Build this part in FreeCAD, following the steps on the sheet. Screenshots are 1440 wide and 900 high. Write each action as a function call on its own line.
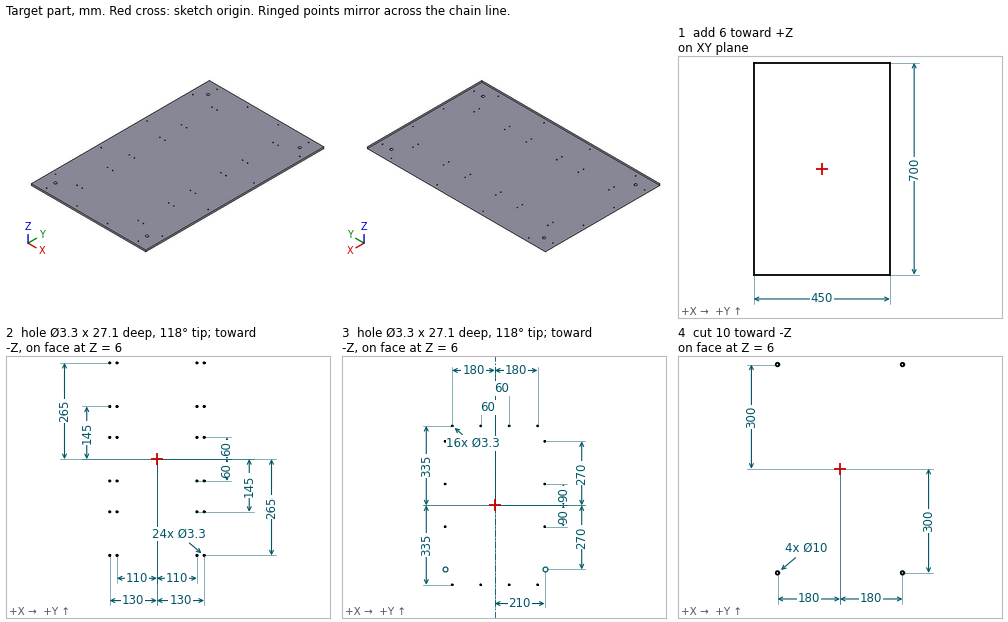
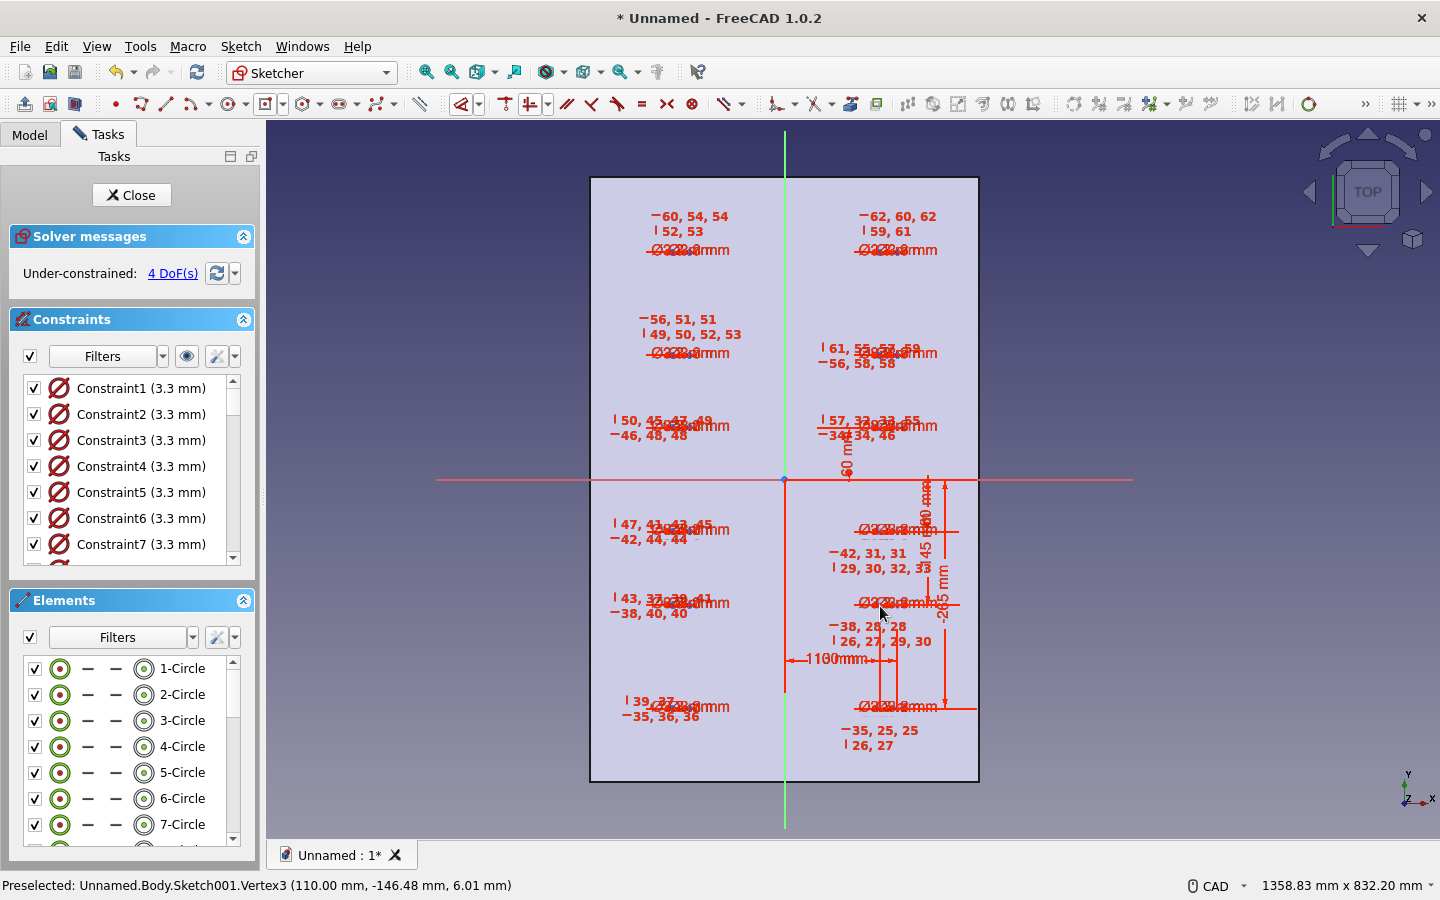
click(672, 709)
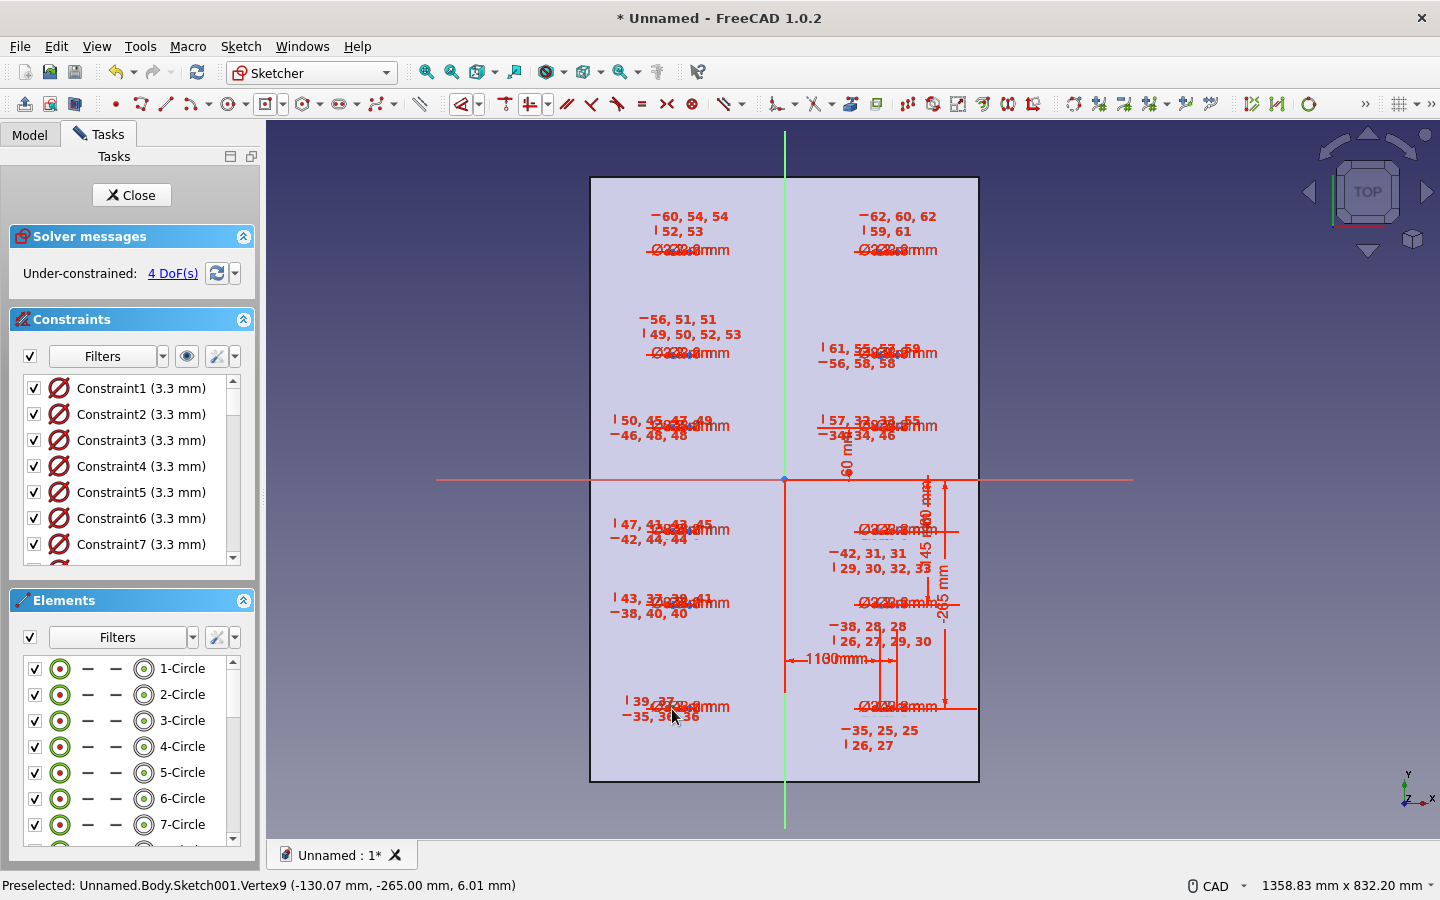
click(478, 104)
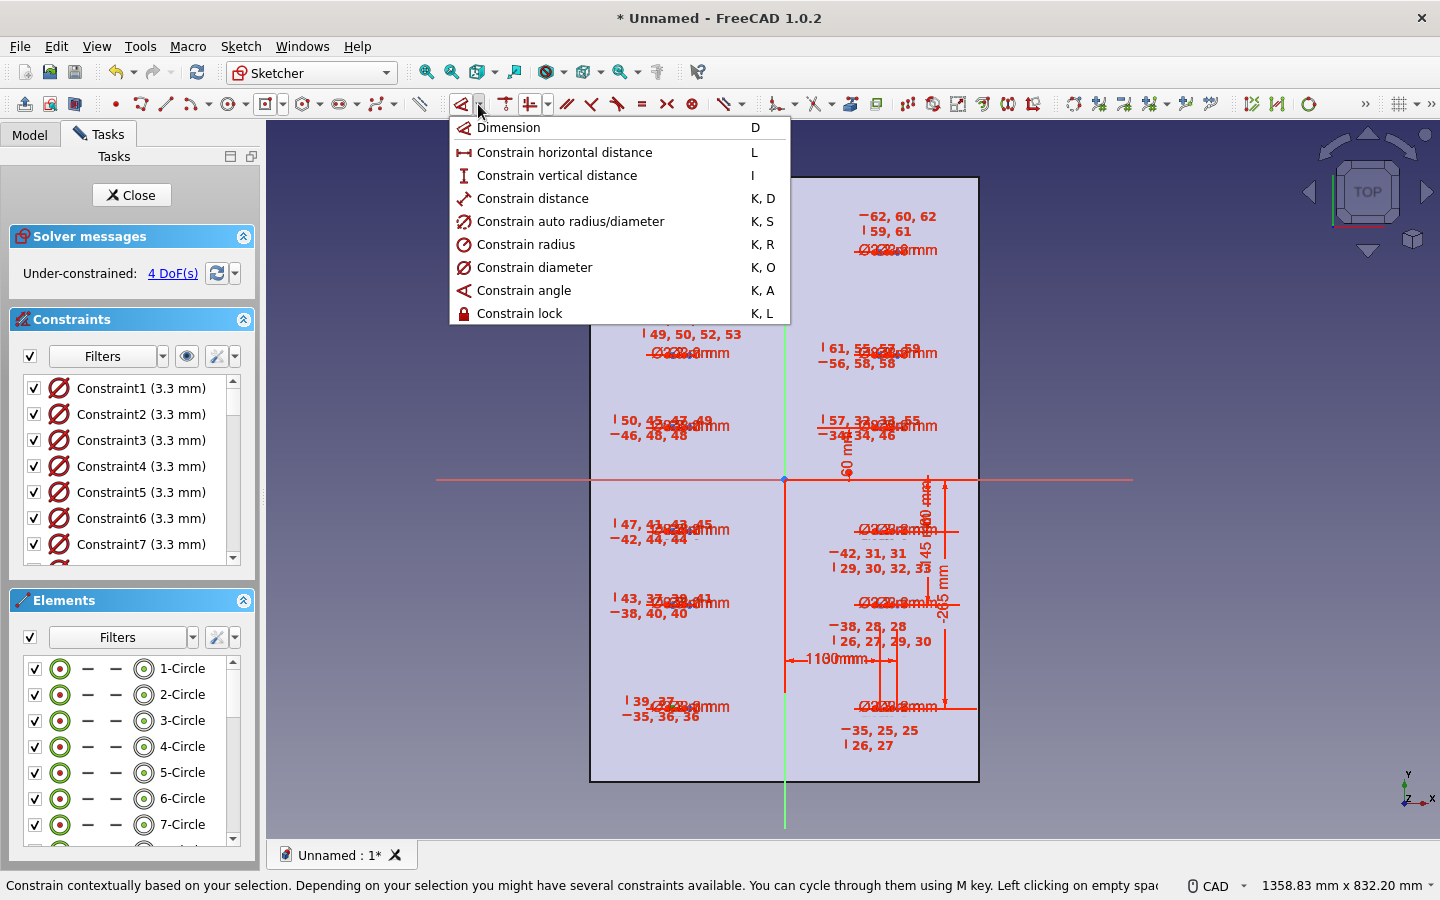
click(620, 152)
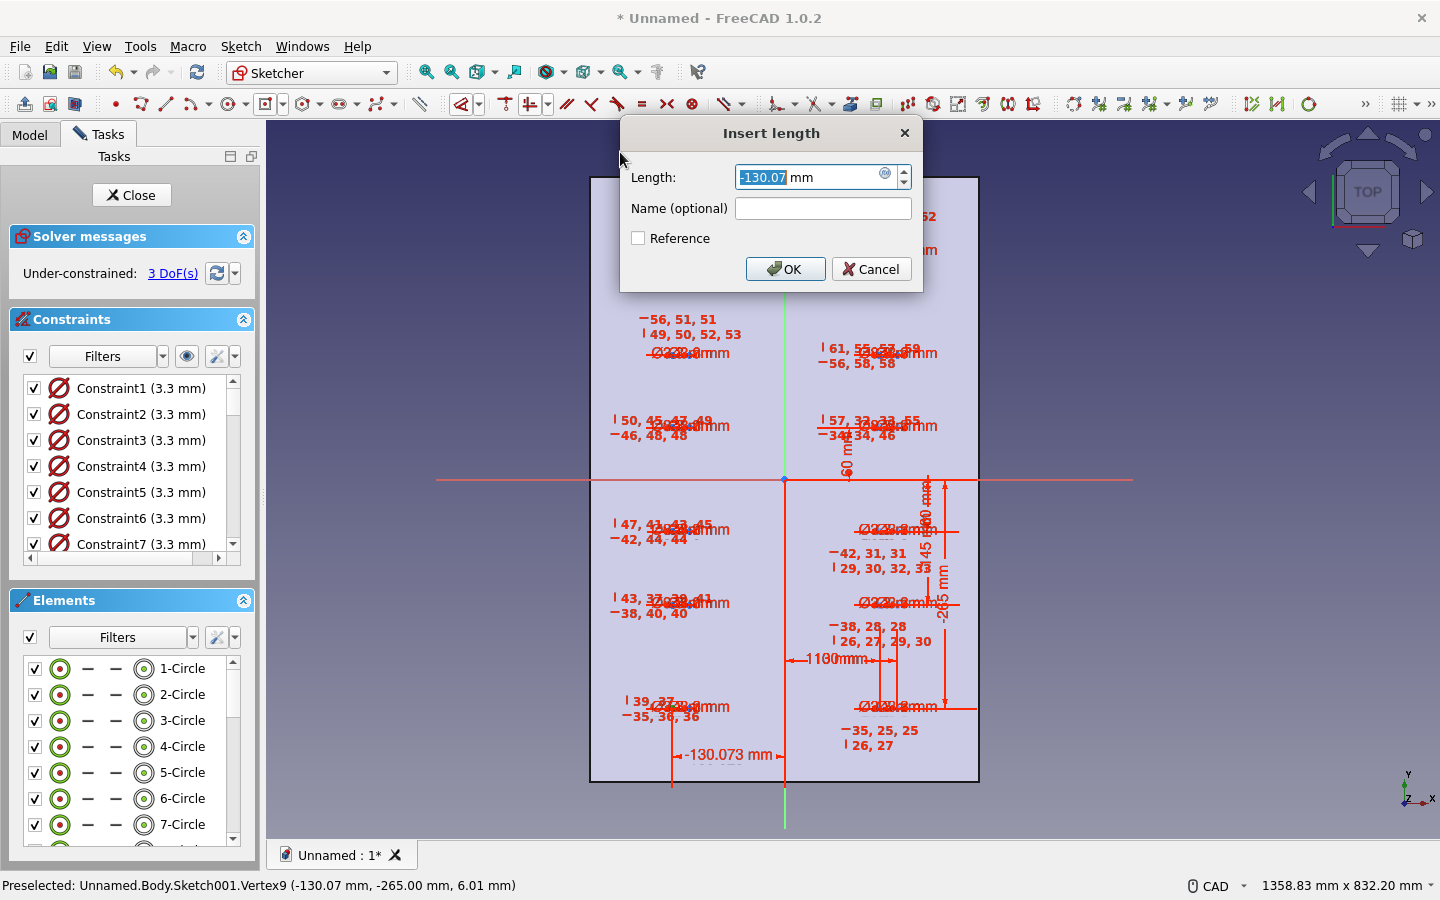
text(-130)
key(Return)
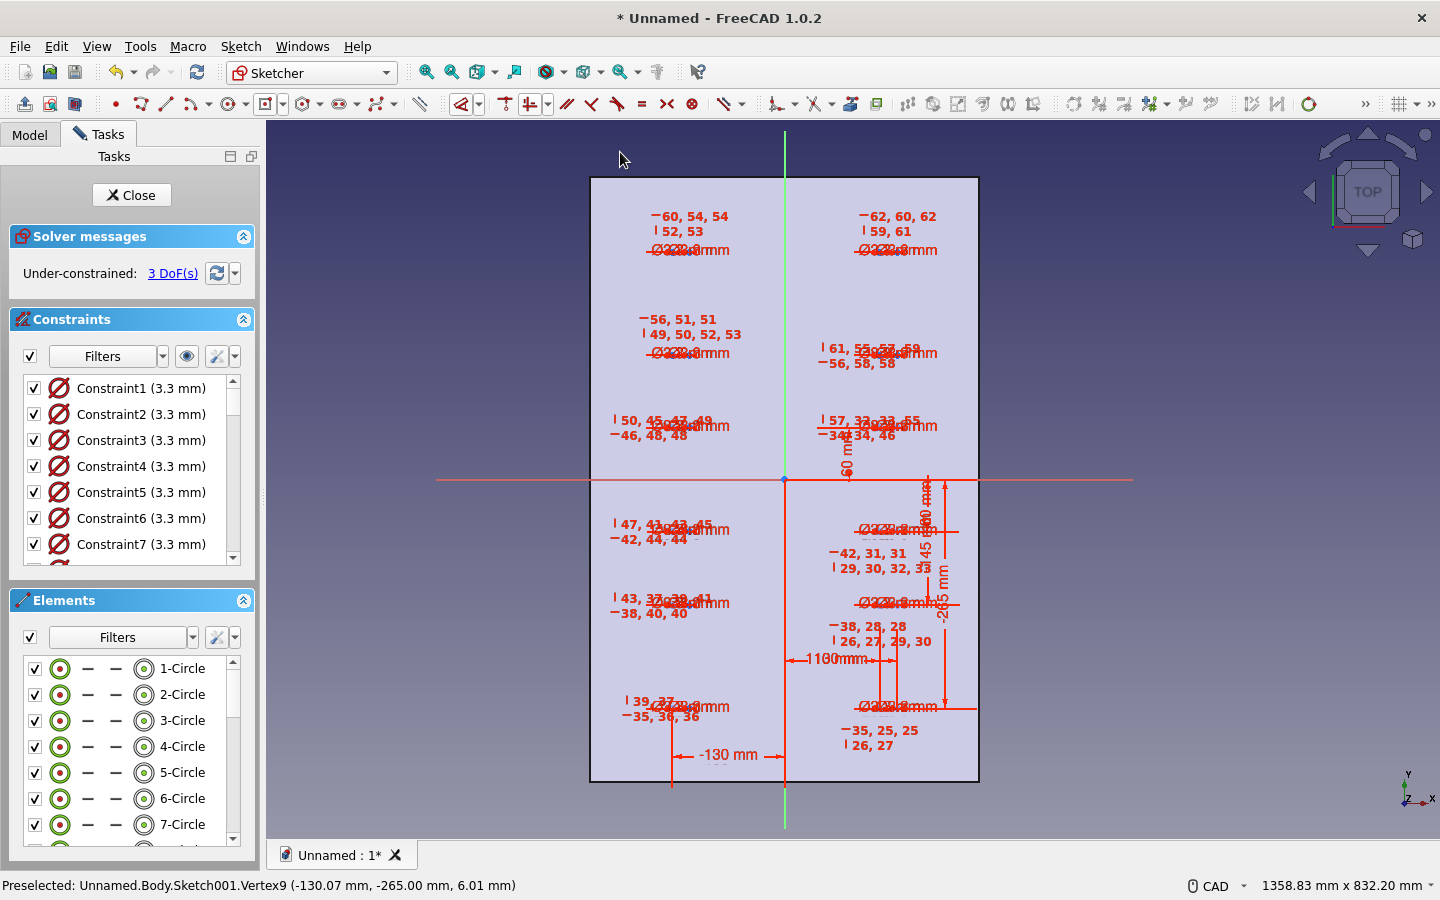
click(689, 709)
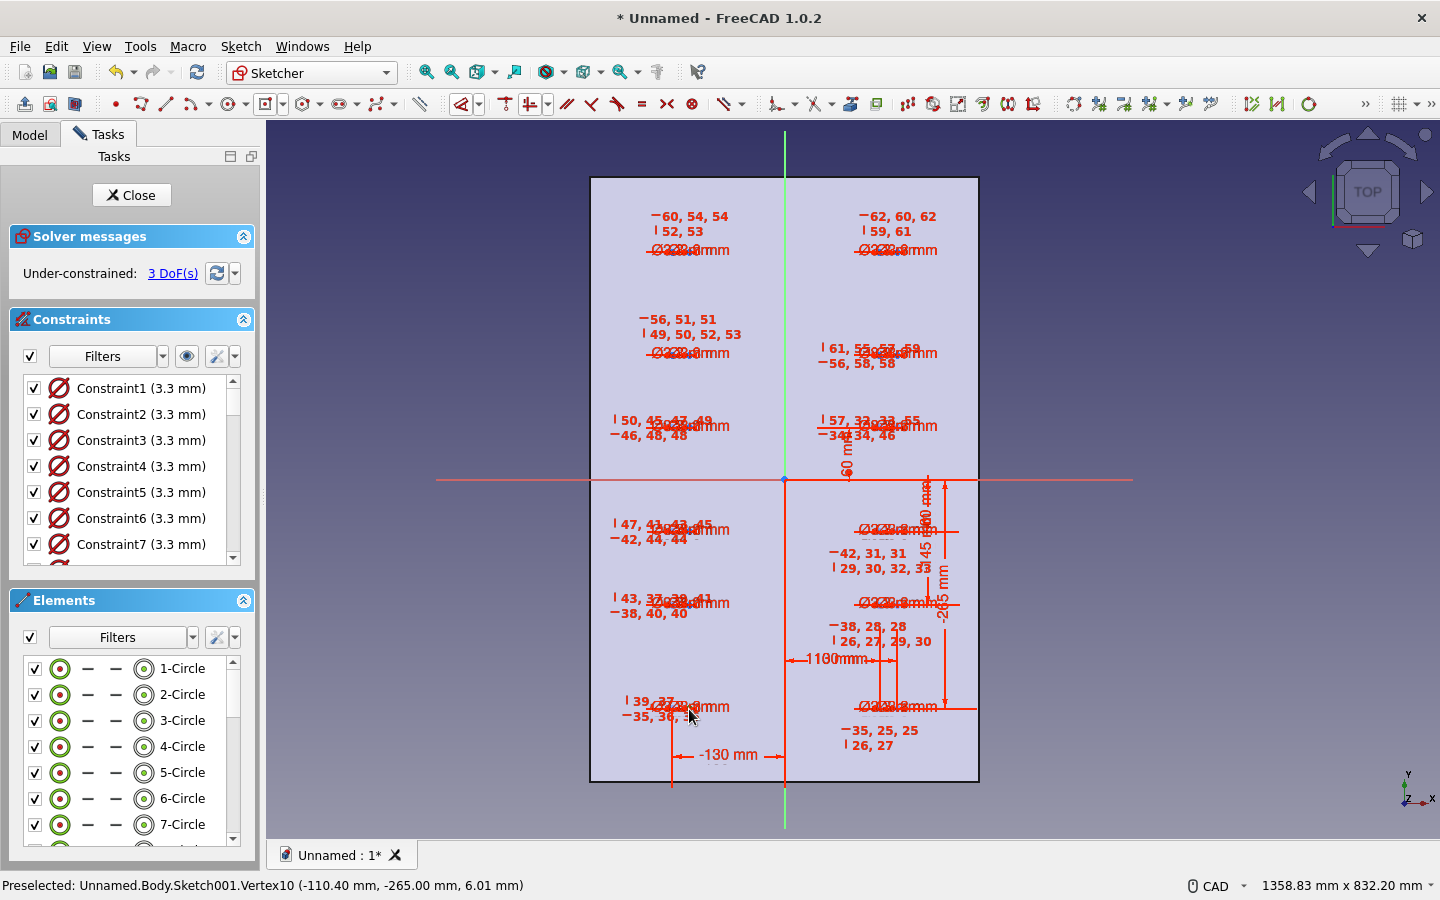
click(478, 104)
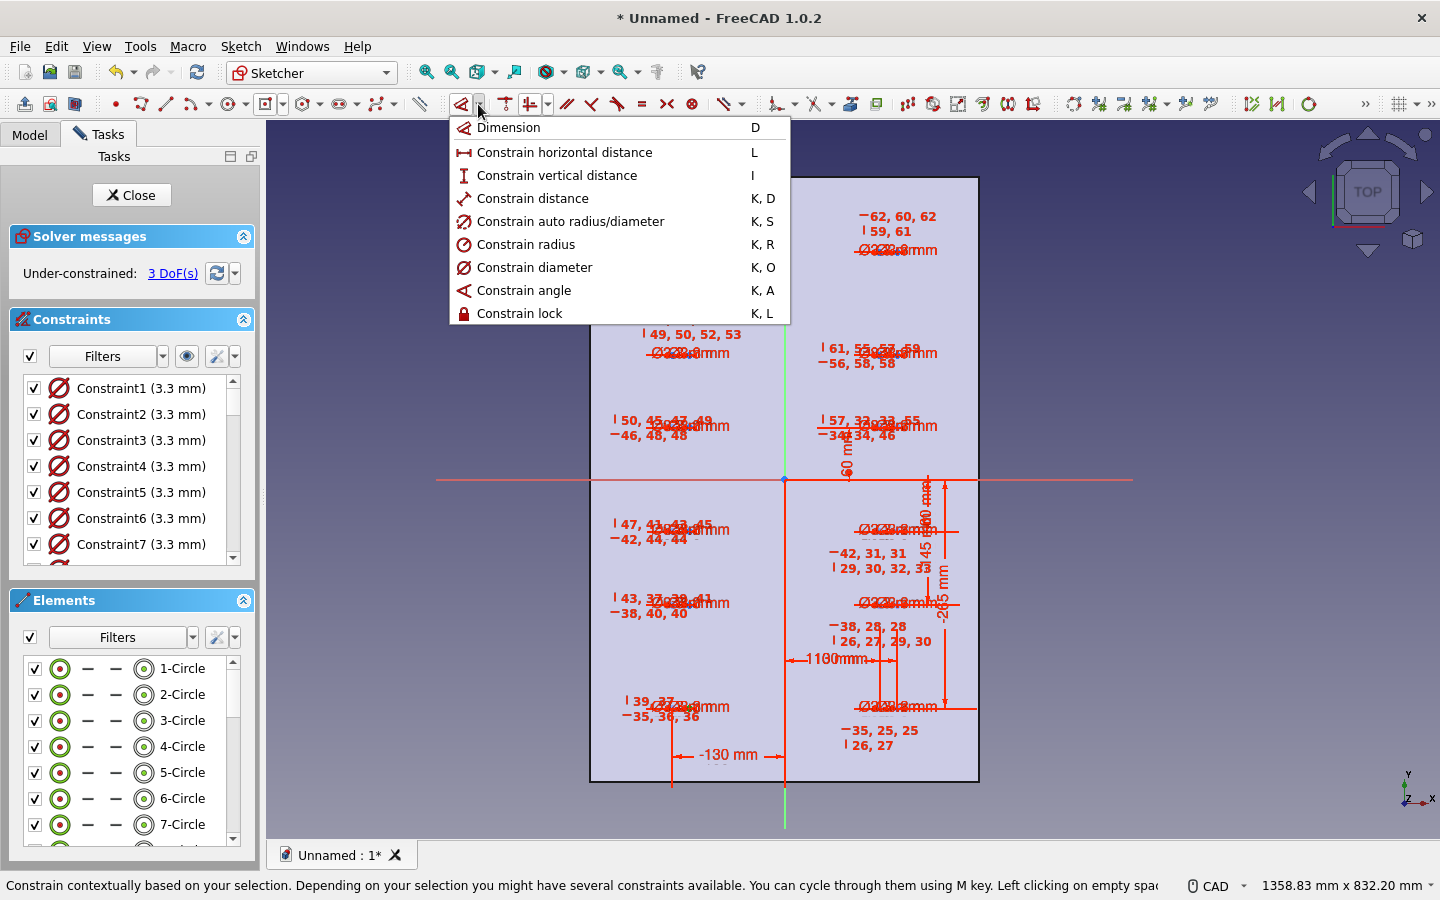
click(620, 152)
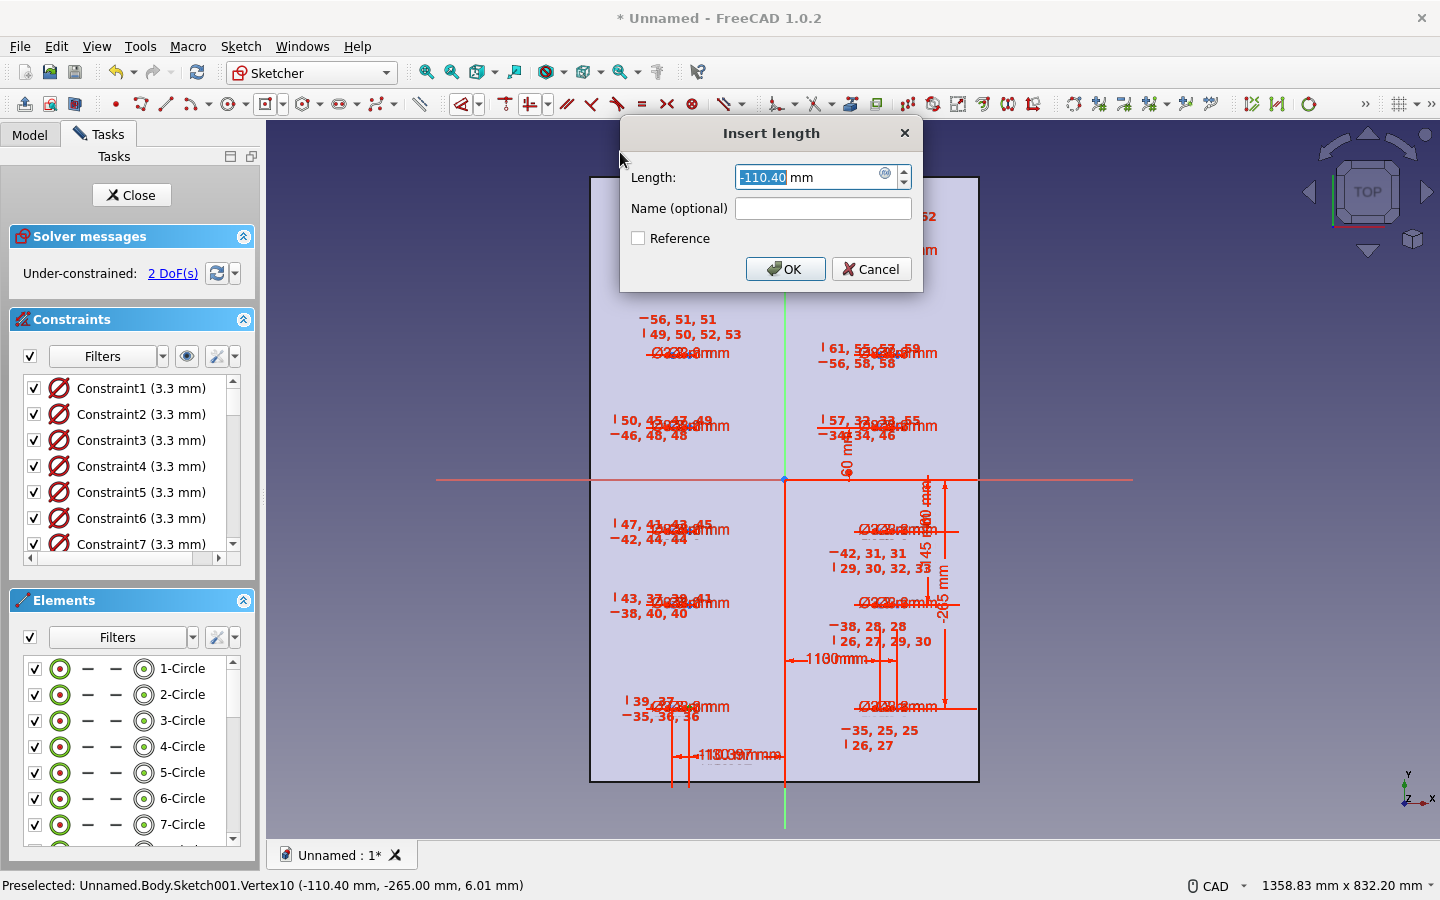
text(-110)
key(Return)